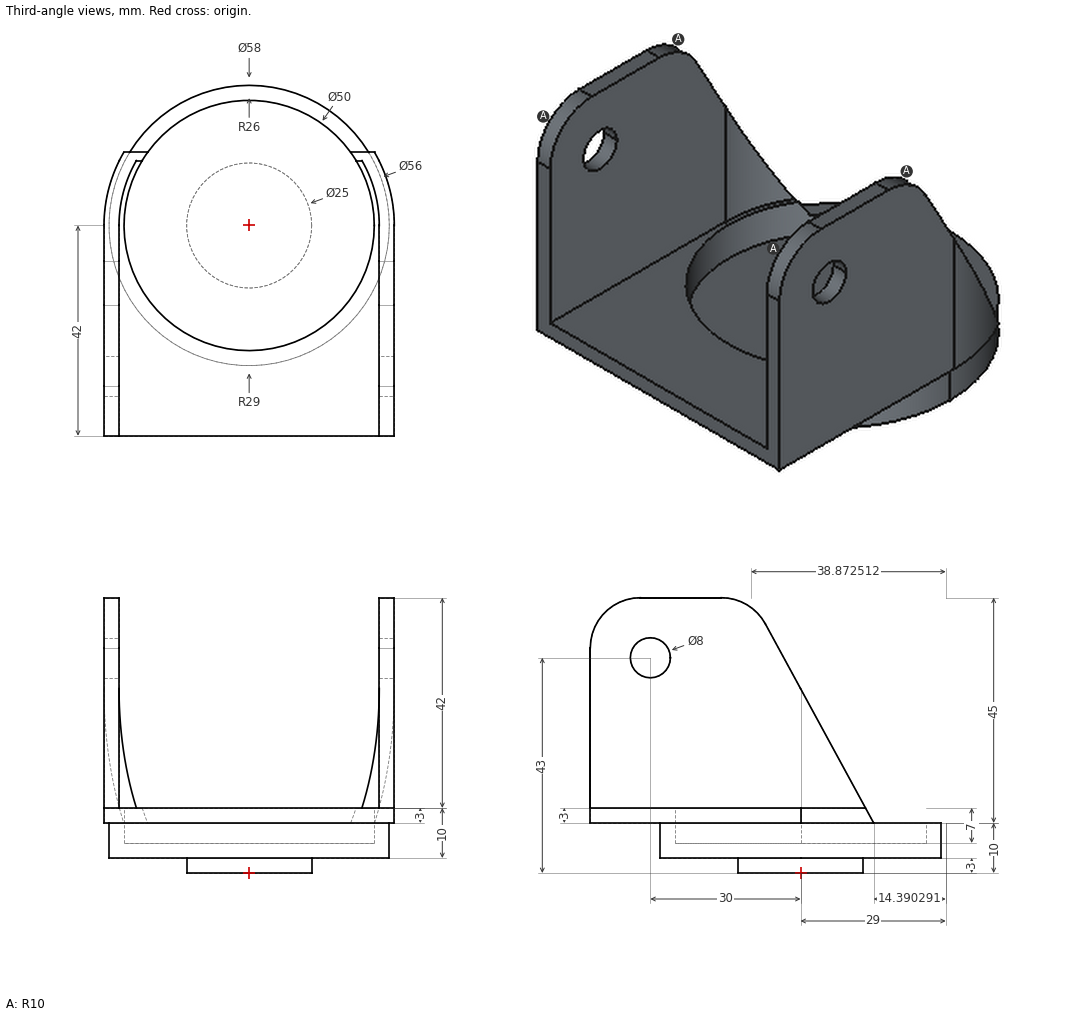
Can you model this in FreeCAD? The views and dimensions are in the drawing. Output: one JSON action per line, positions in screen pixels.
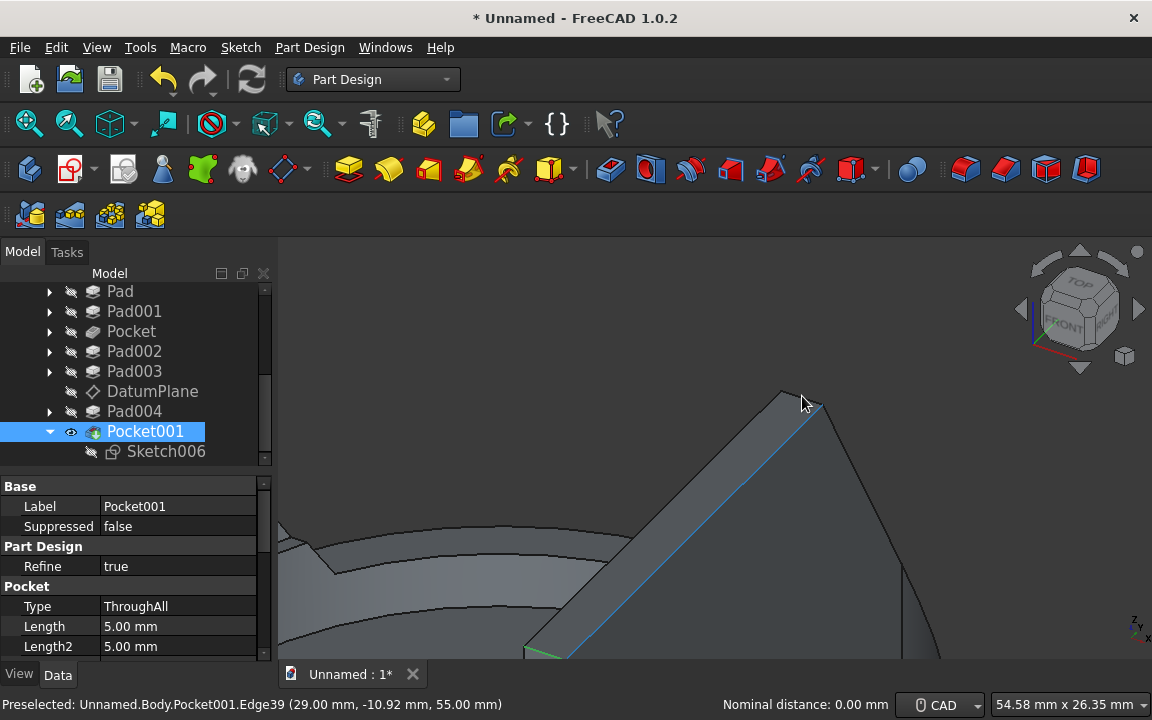
{"action": "left_click", "coordinate": [30, 124]}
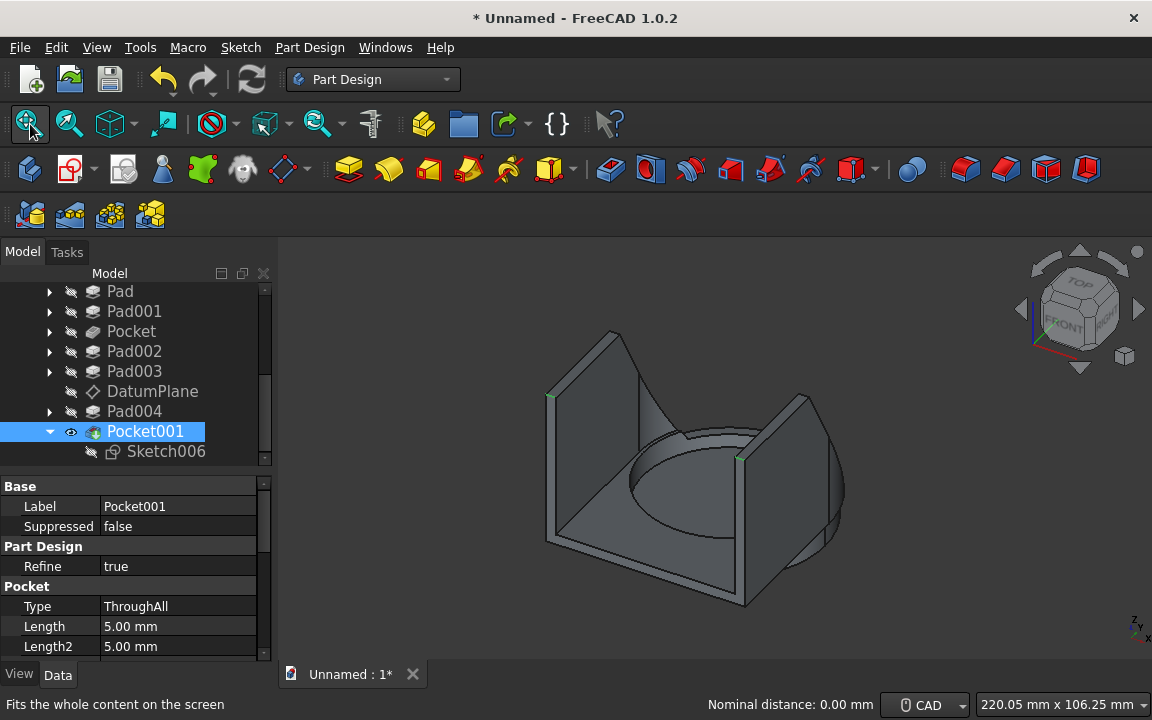
{"action": "key", "text": "0"}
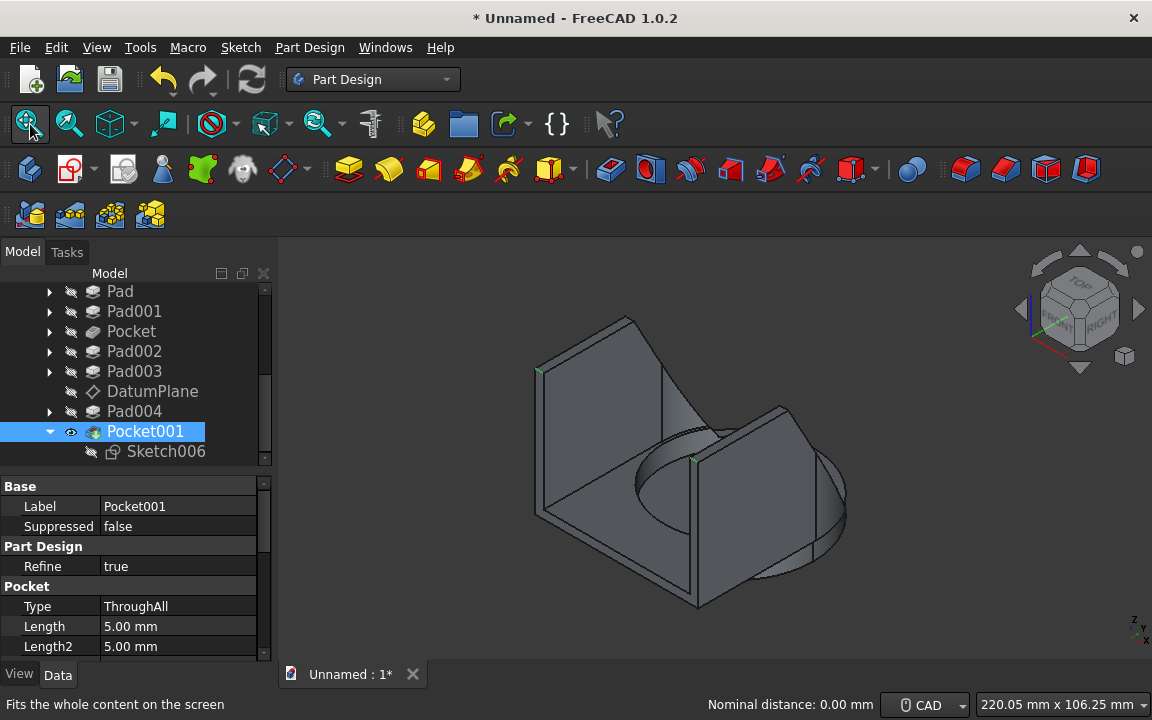
{"action": "scroll", "coordinate": [784, 407], "scroll_direction": "up", "scroll_amount": 7}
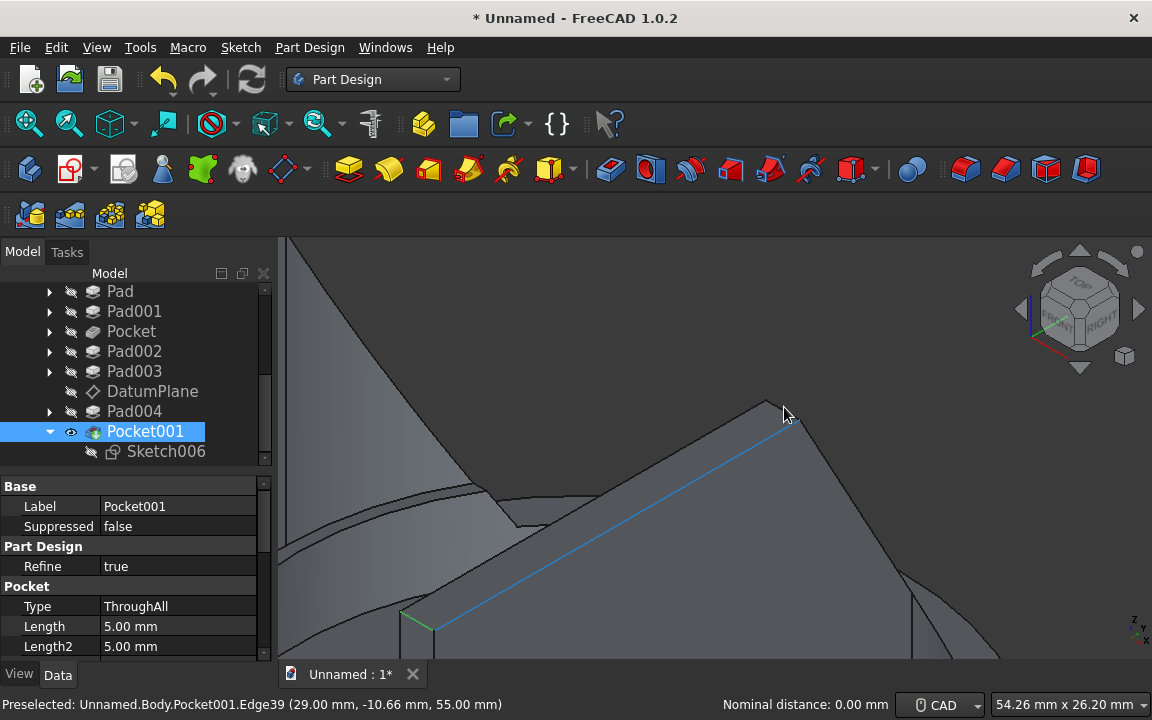
{"action": "left_click", "coordinate": [30, 124]}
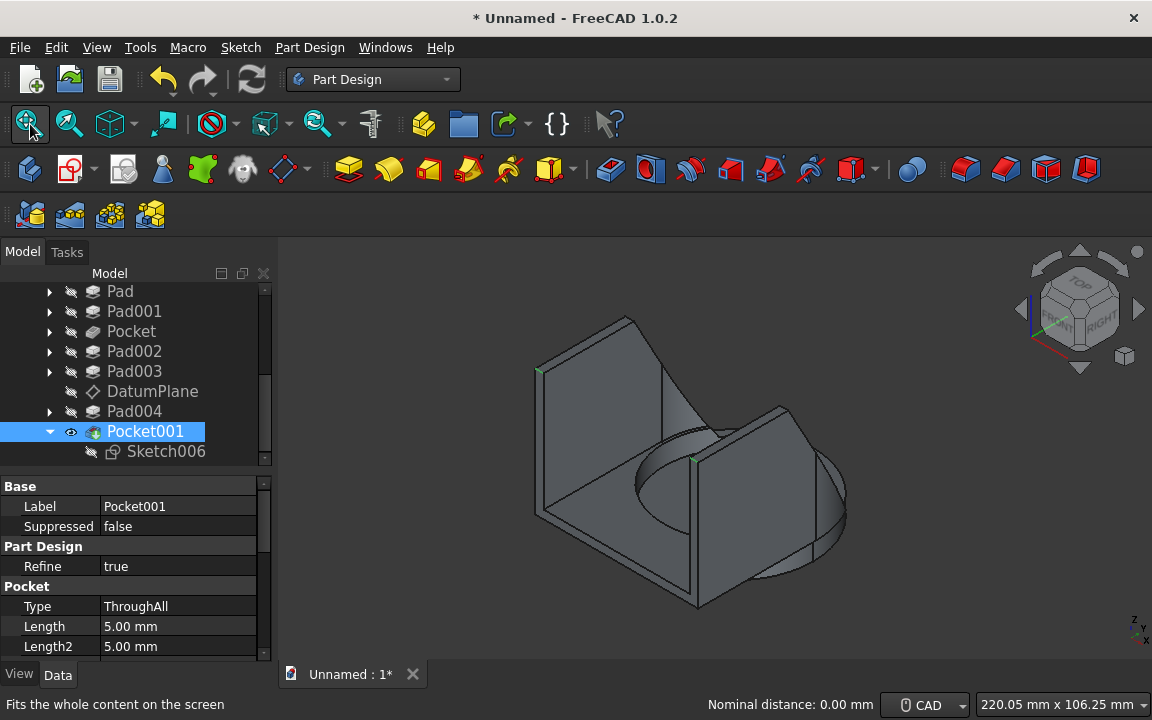
{"action": "key", "text": "2"}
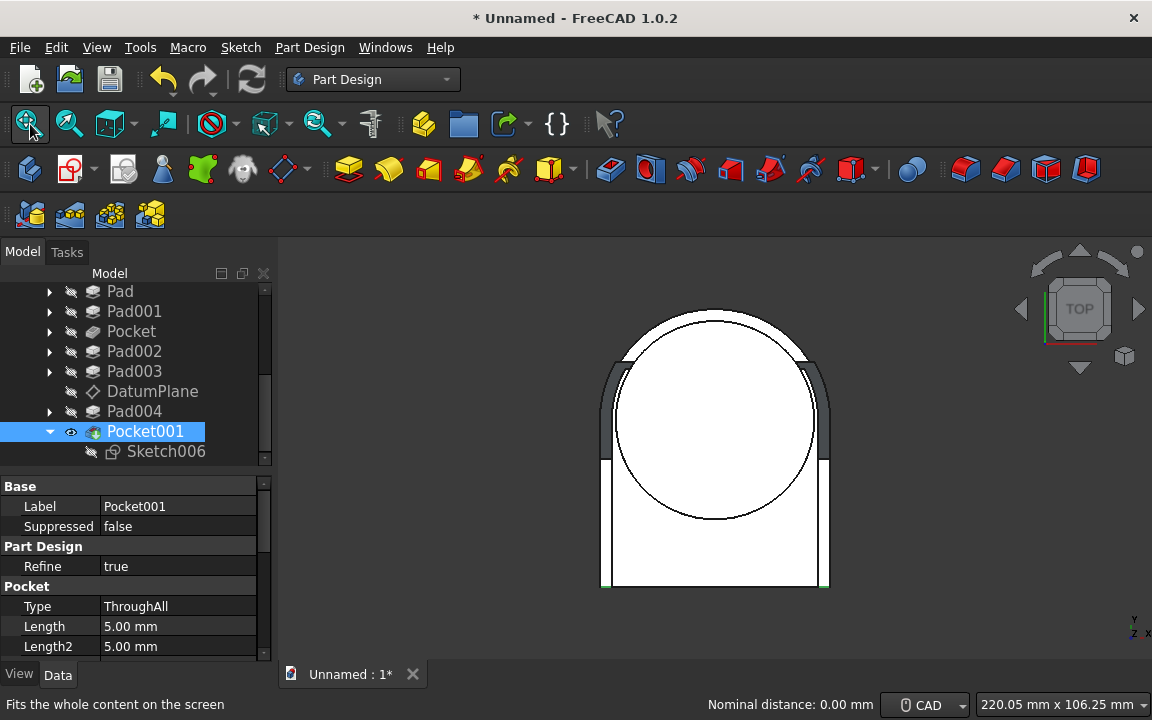
{"action": "scroll", "coordinate": [824, 458], "scroll_direction": "up", "scroll_amount": 7}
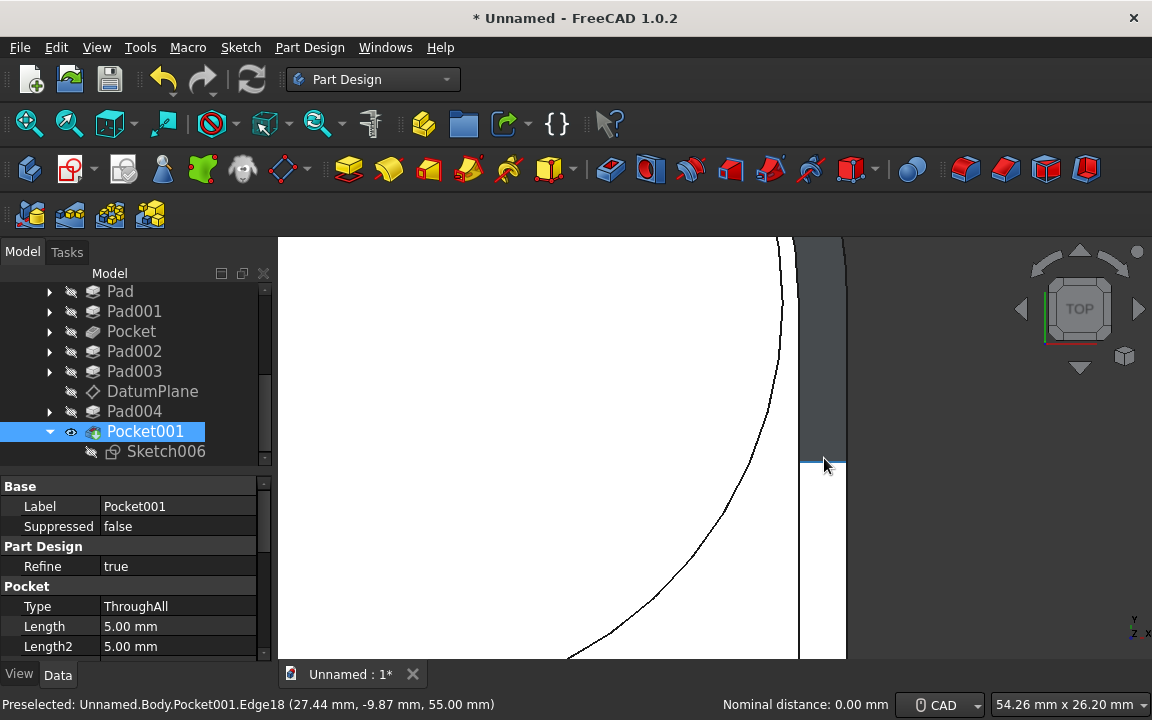
{"action": "left_click", "coordinate": [823, 461], "text": "ctrl"}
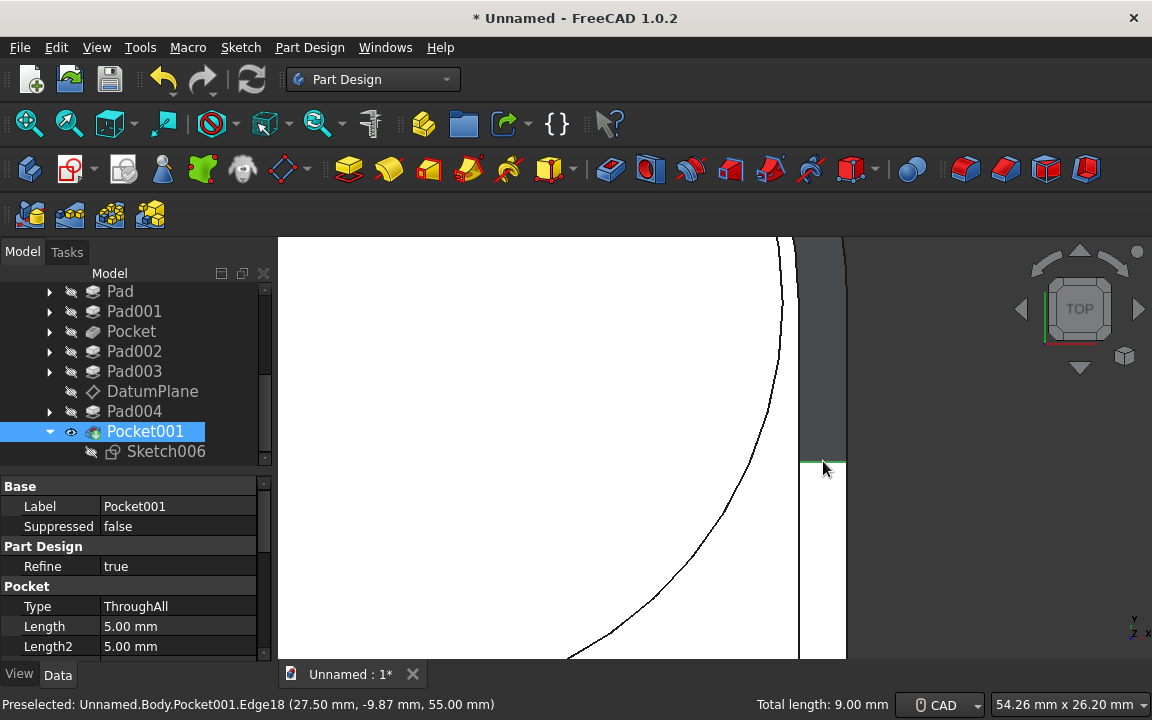
{"action": "left_click", "coordinate": [30, 124]}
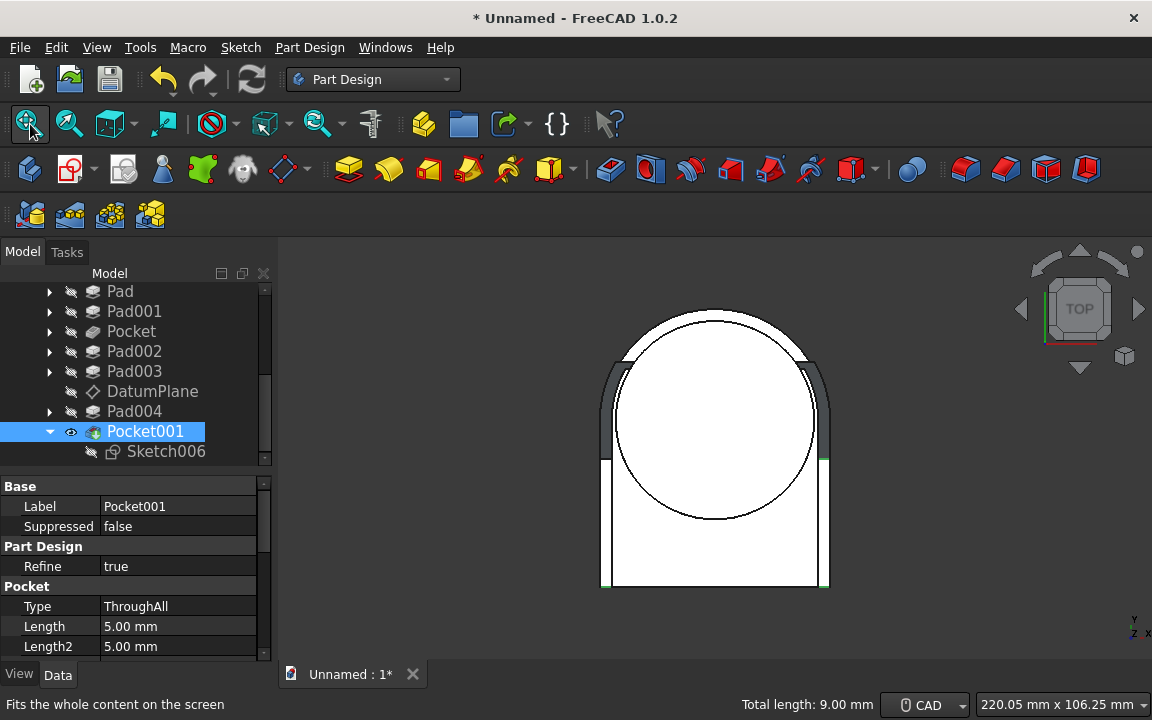
{"action": "key", "text": "1"}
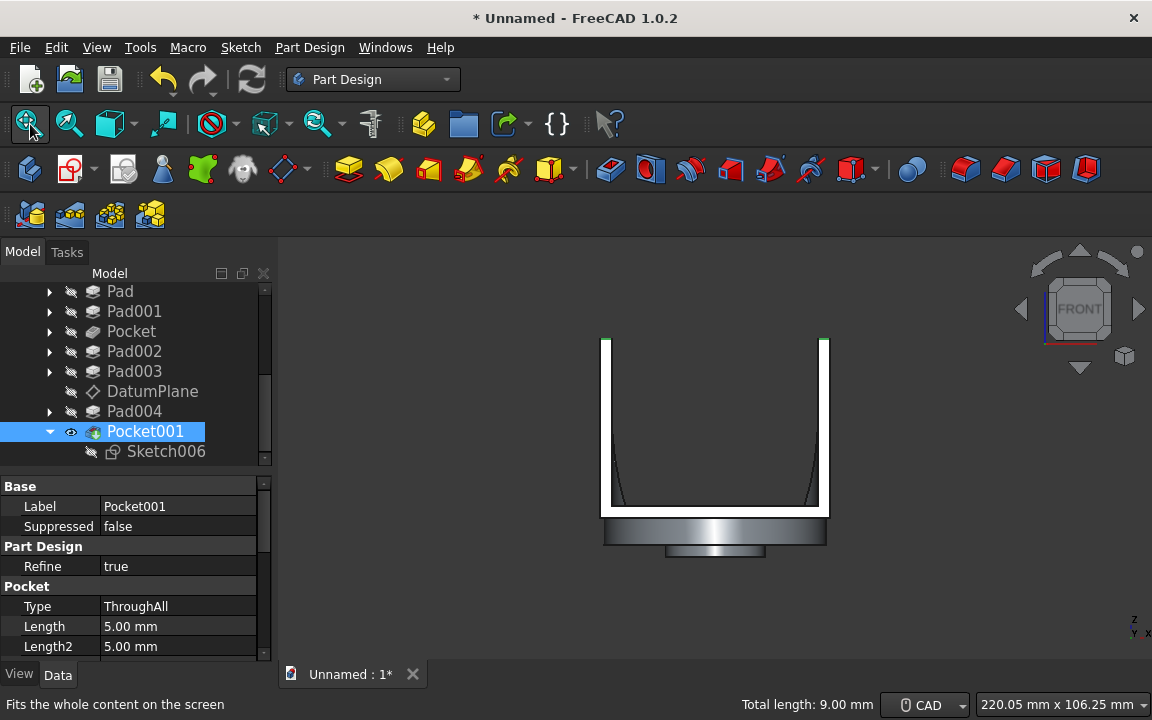
{"action": "scroll", "coordinate": [606, 338], "scroll_direction": "up", "scroll_amount": 7}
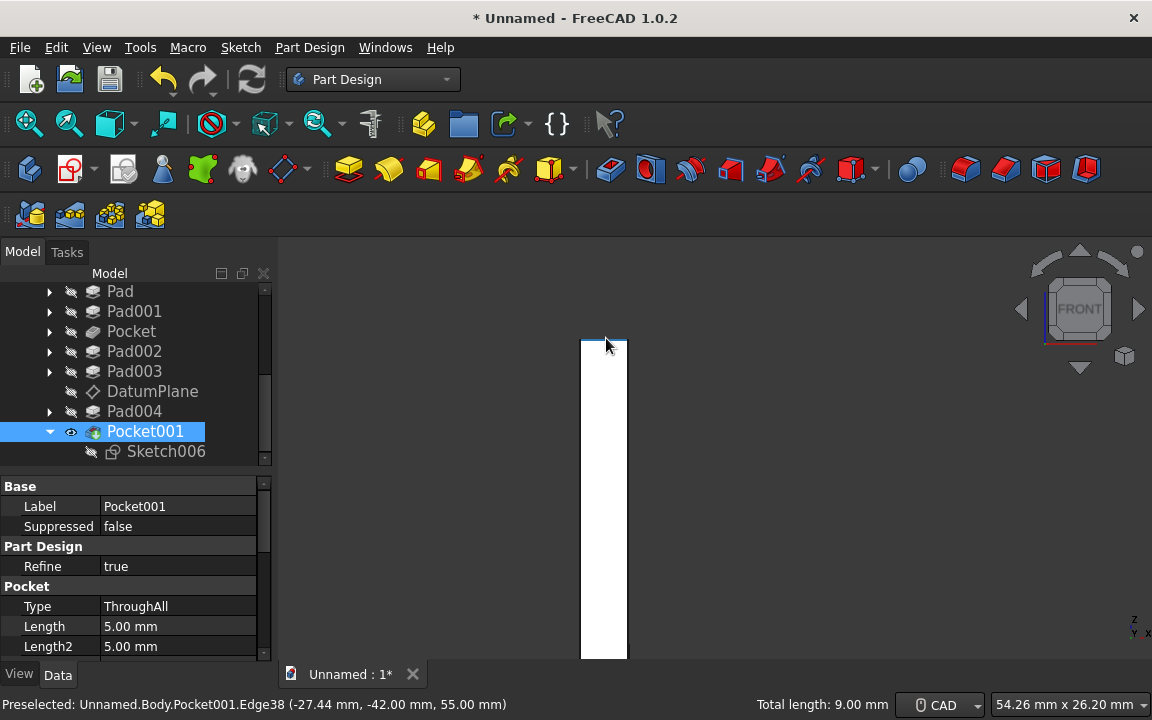
{"action": "left_click", "coordinate": [30, 124]}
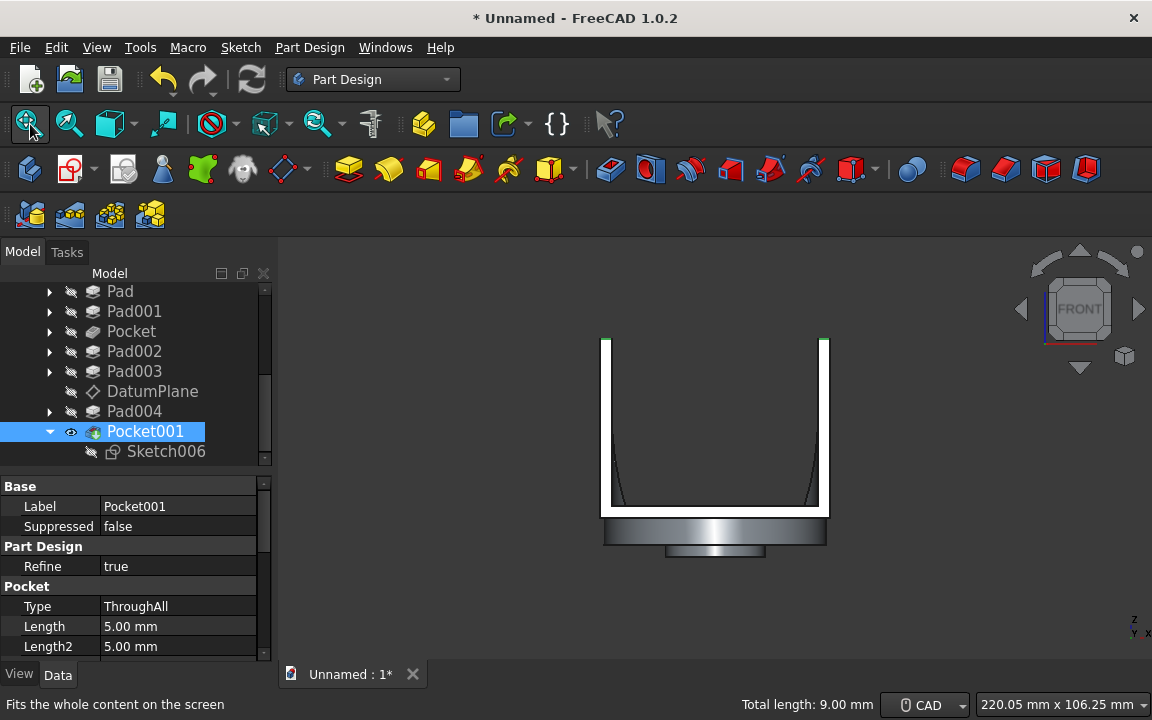
{"action": "key", "text": "3"}